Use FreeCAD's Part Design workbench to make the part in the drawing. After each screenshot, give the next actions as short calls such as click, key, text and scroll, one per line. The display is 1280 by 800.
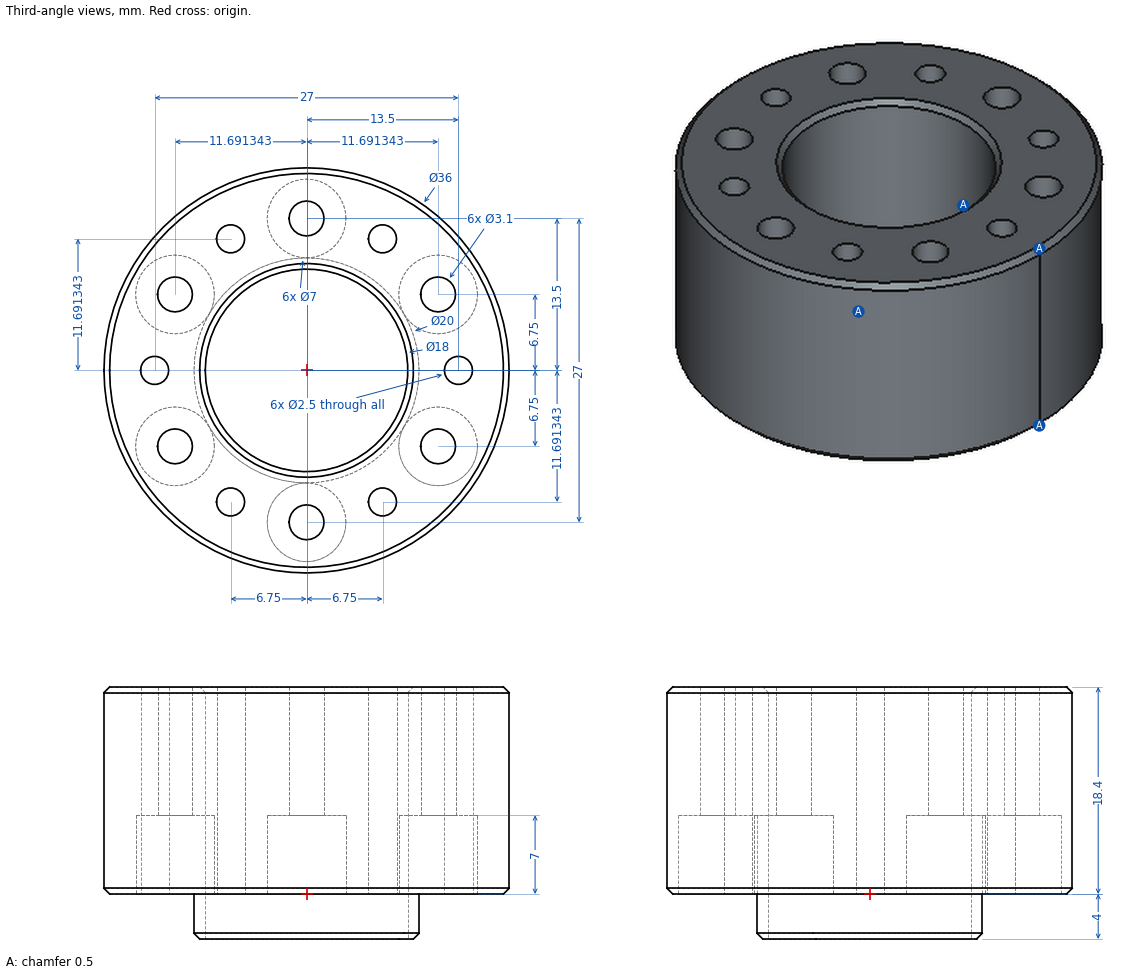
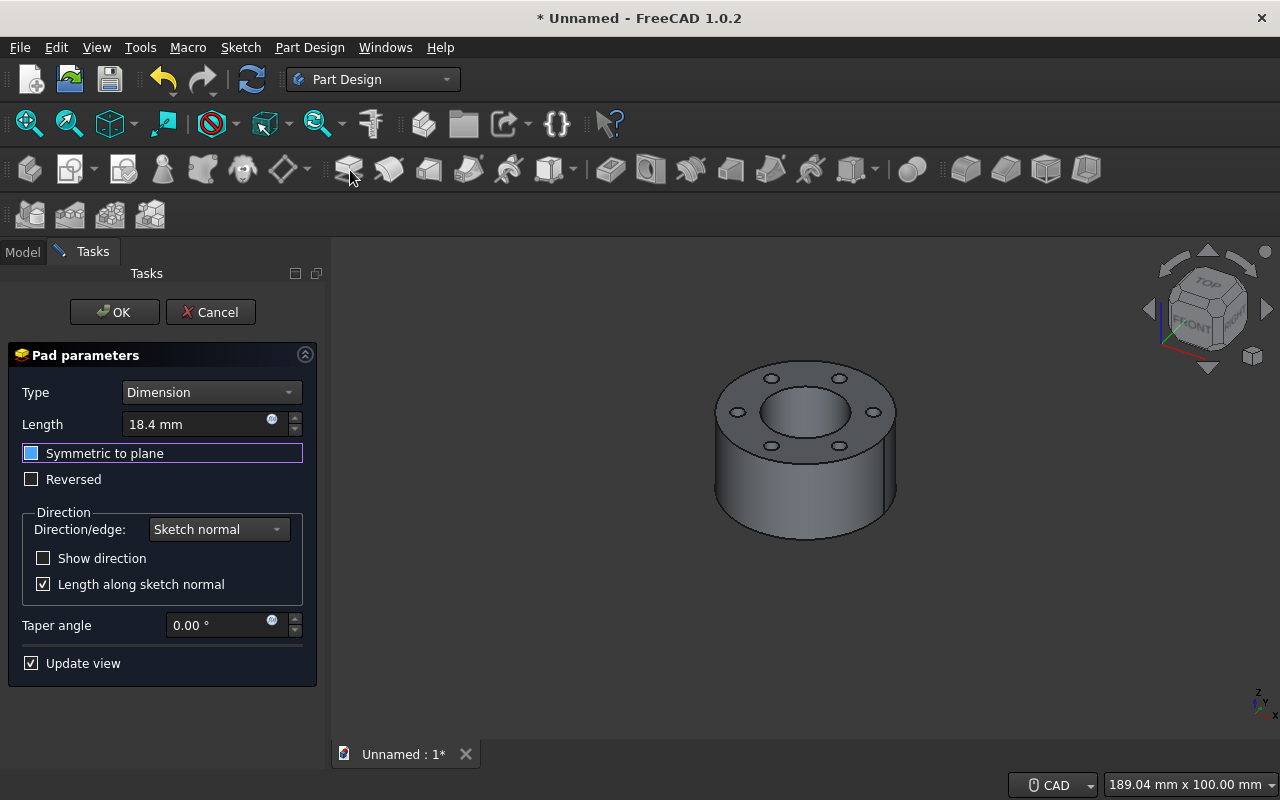
click(115, 312)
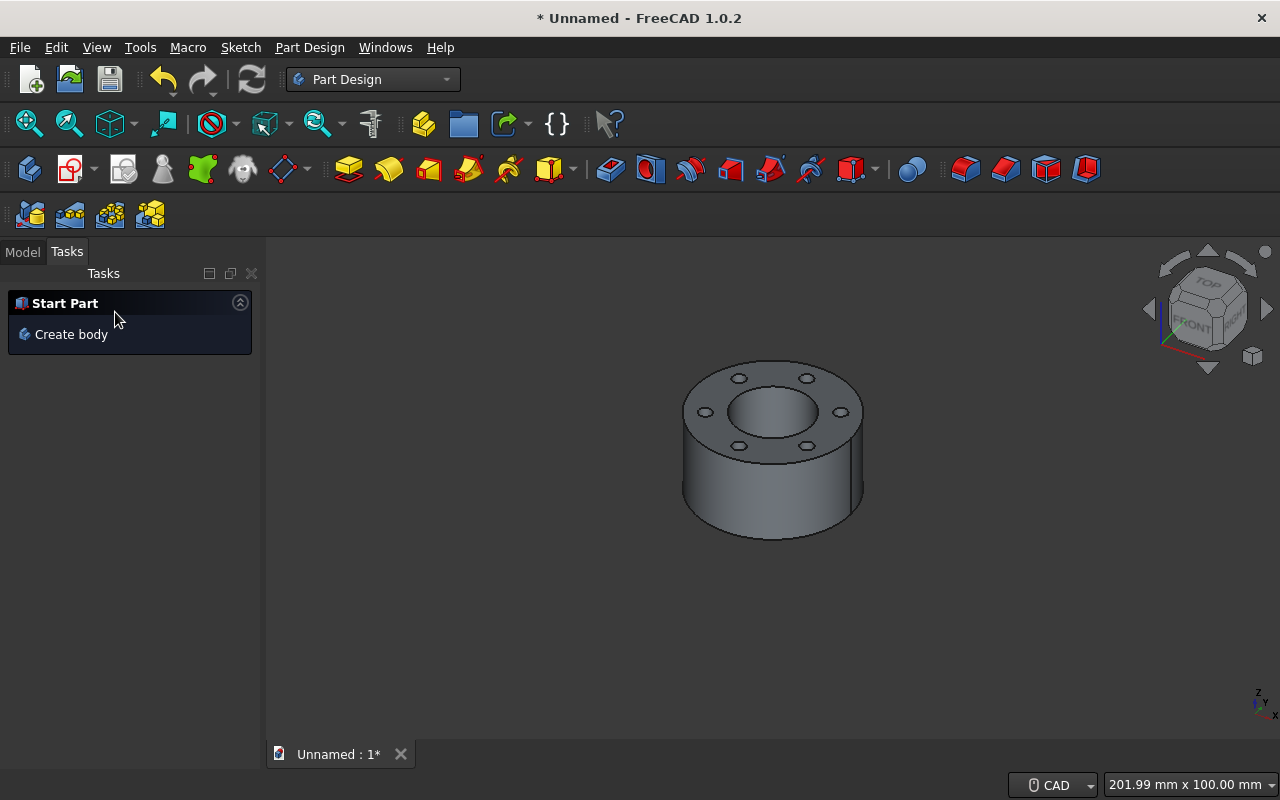
click(30, 124)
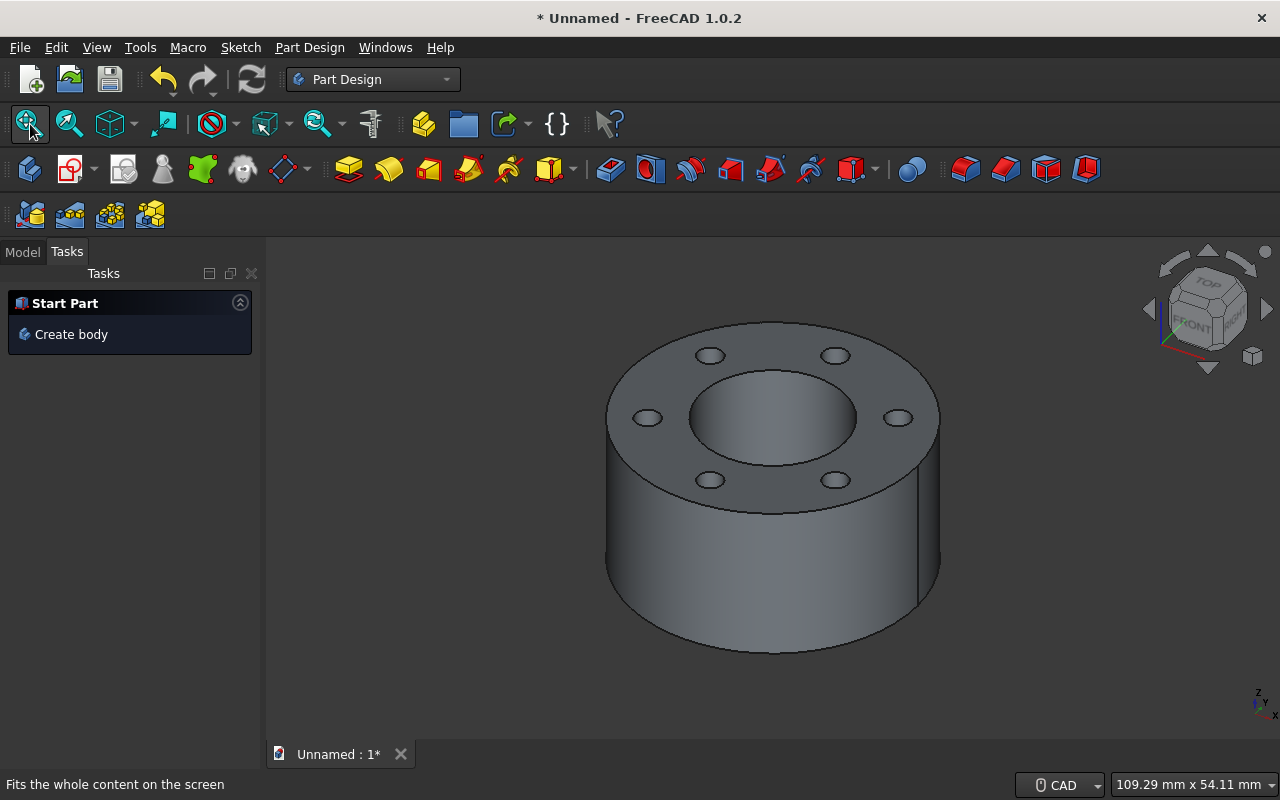
click(70, 170)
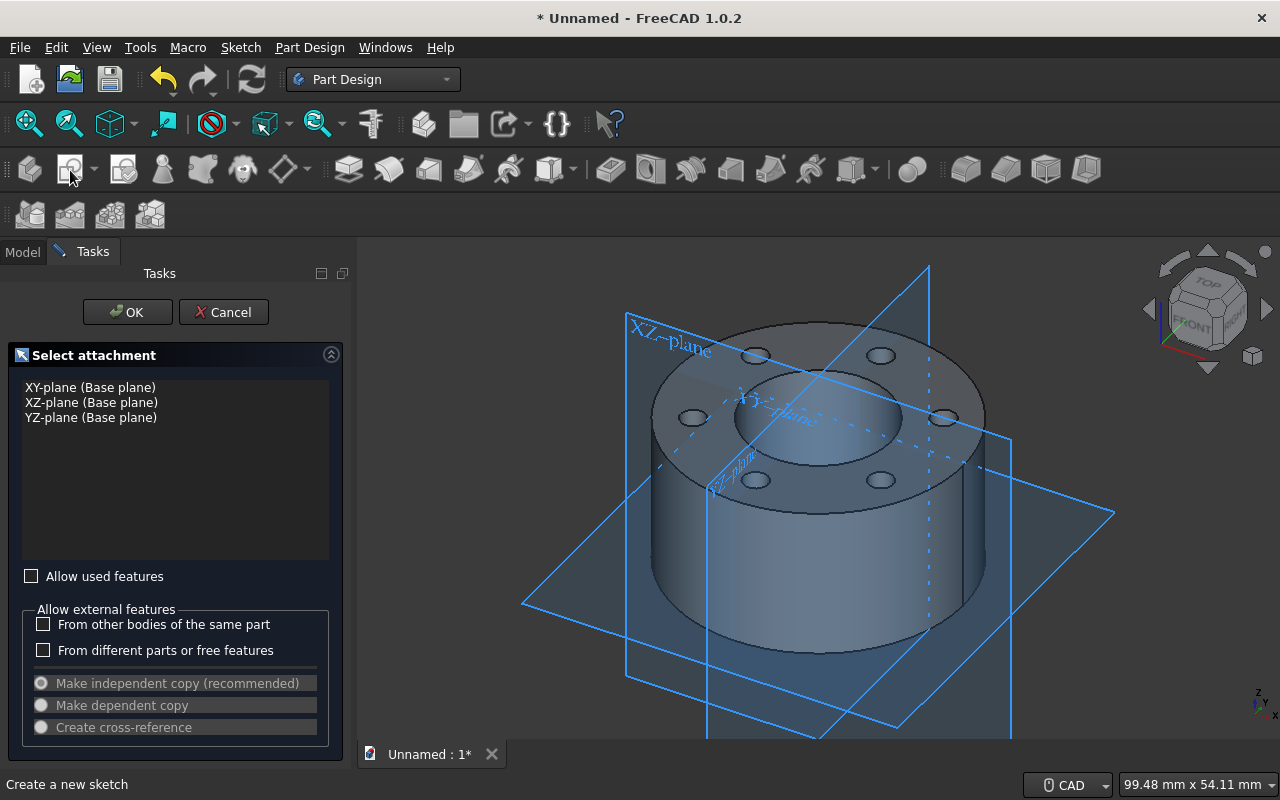
click(82, 388)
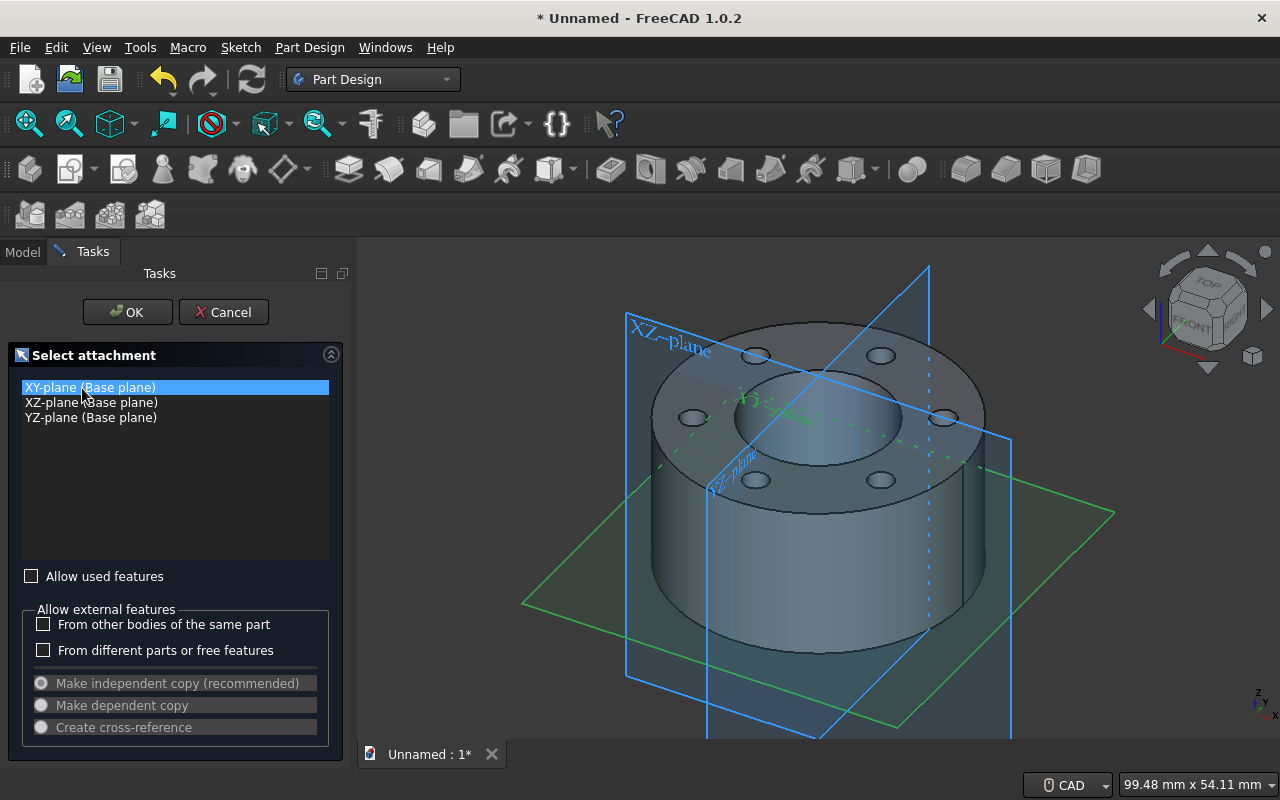
click(128, 312)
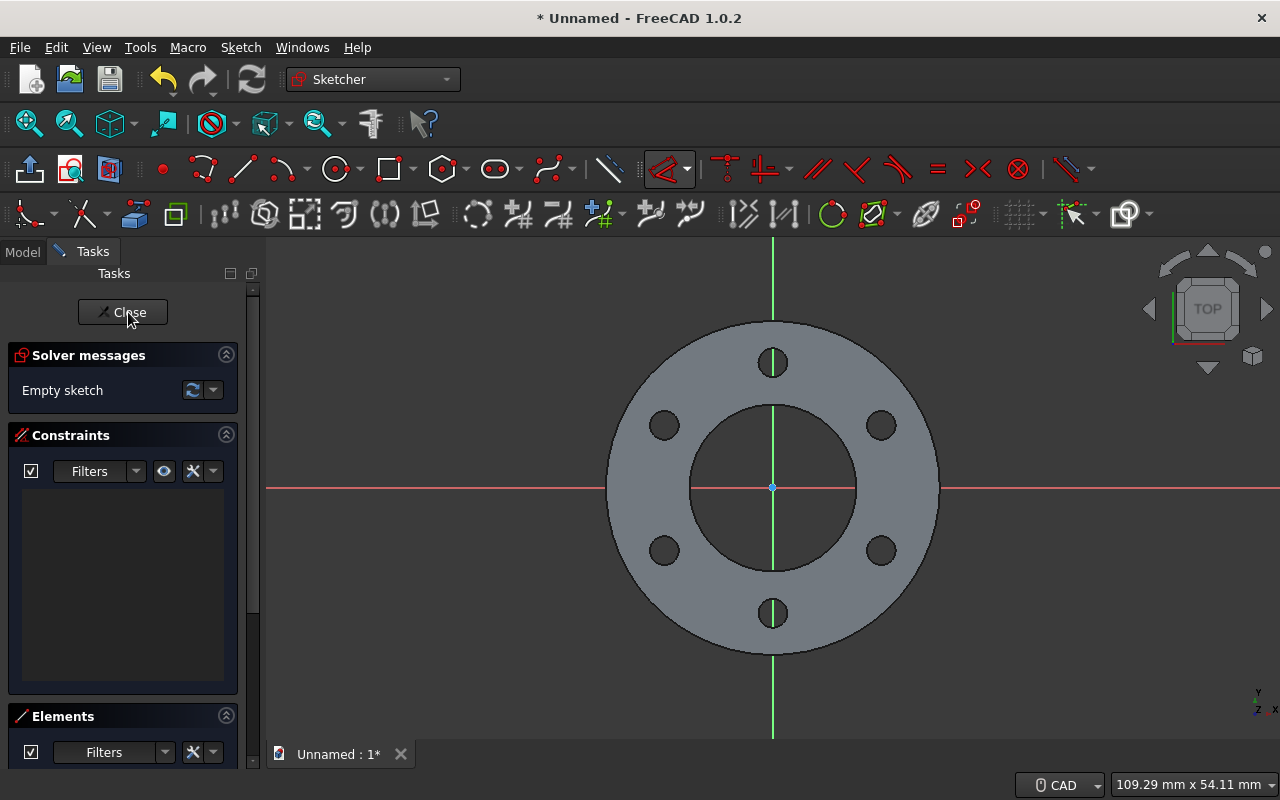
click(110, 170)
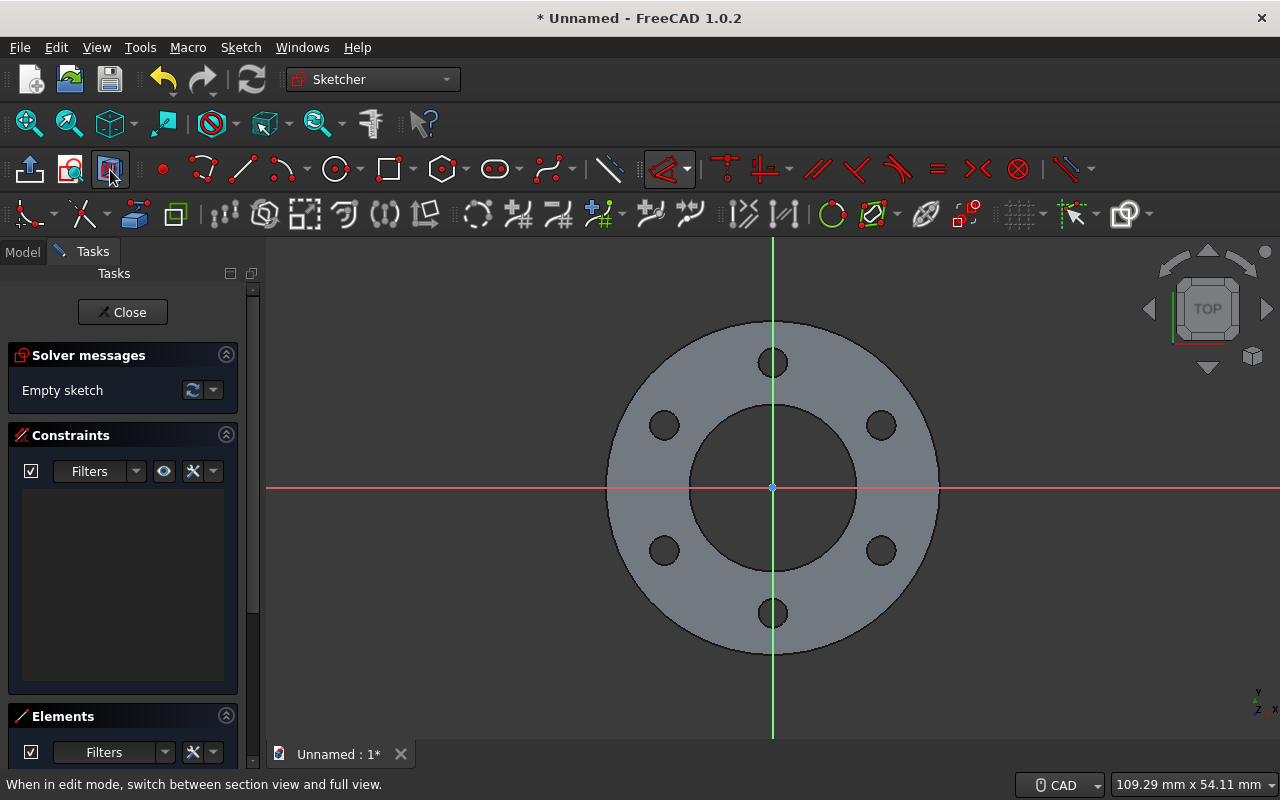
click(336, 170)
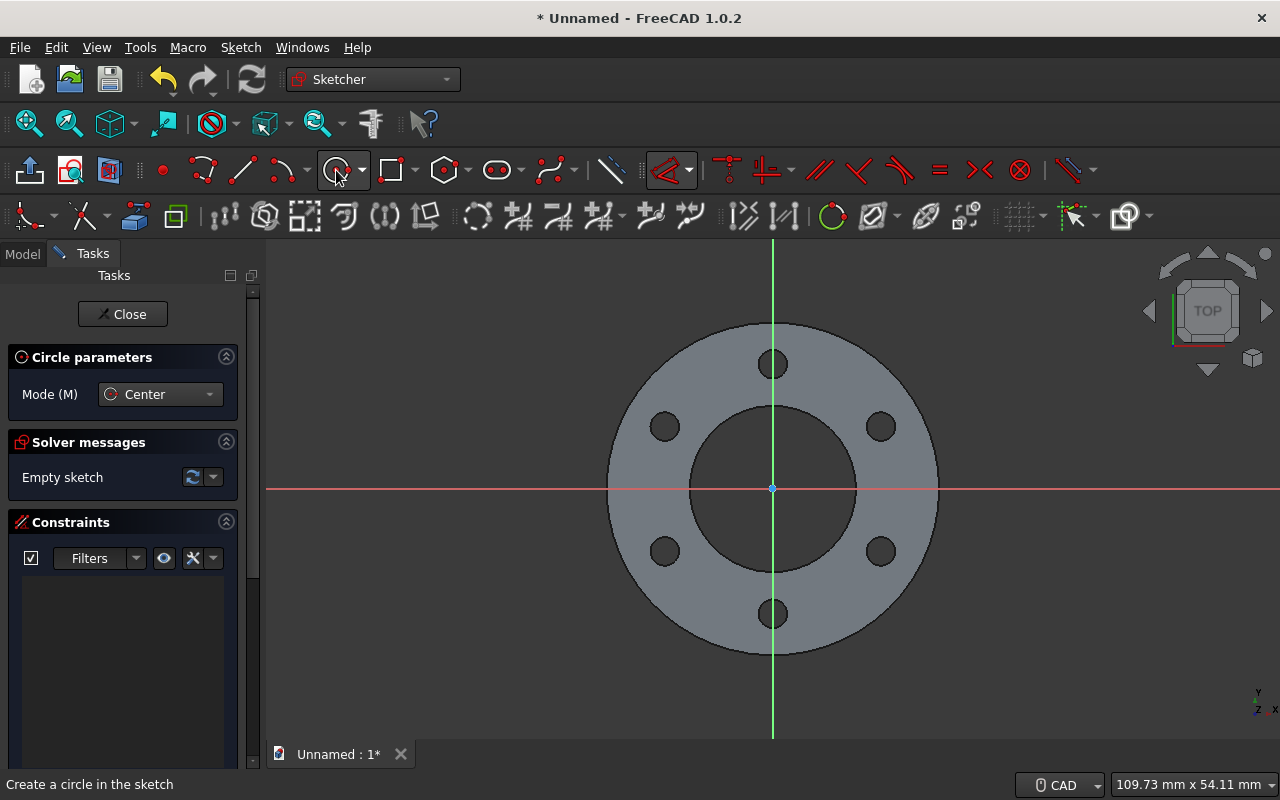
click(773, 364)
click(796, 341)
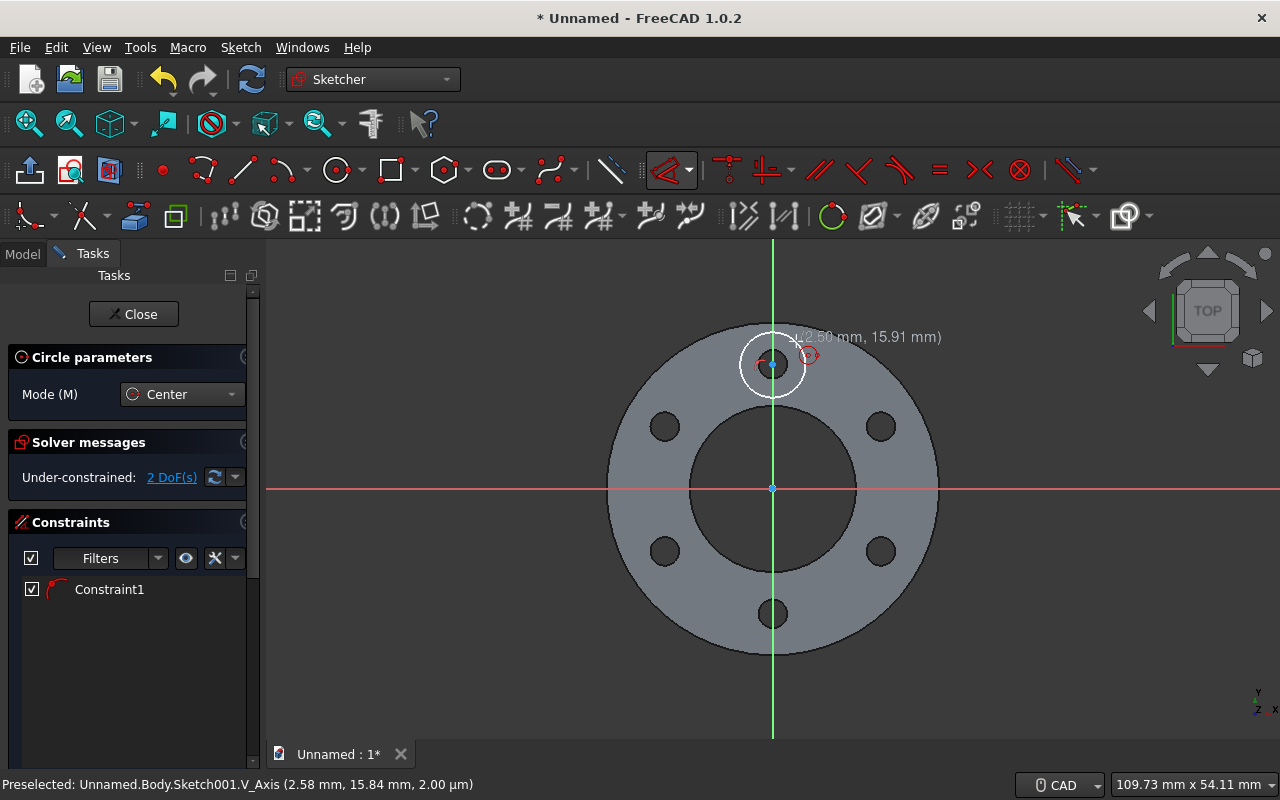
click(881, 427)
click(904, 404)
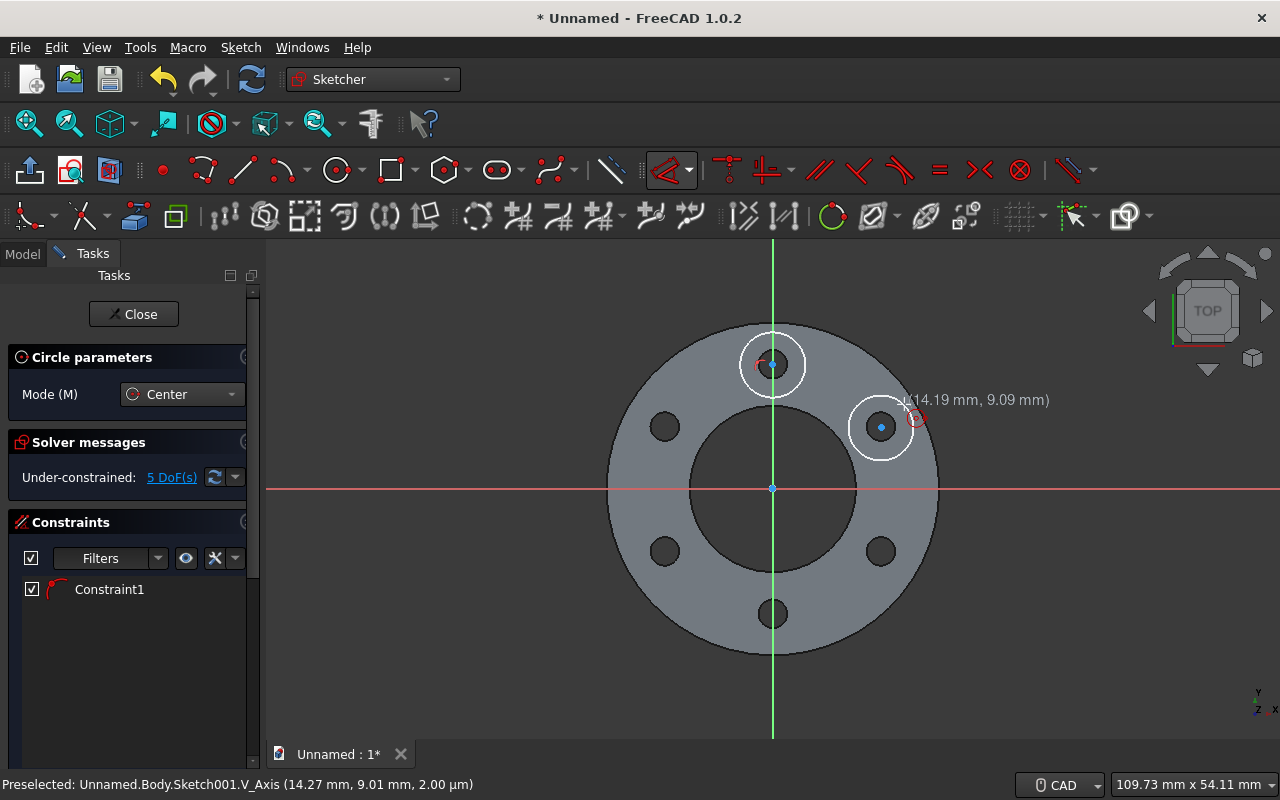
click(881, 551)
click(904, 529)